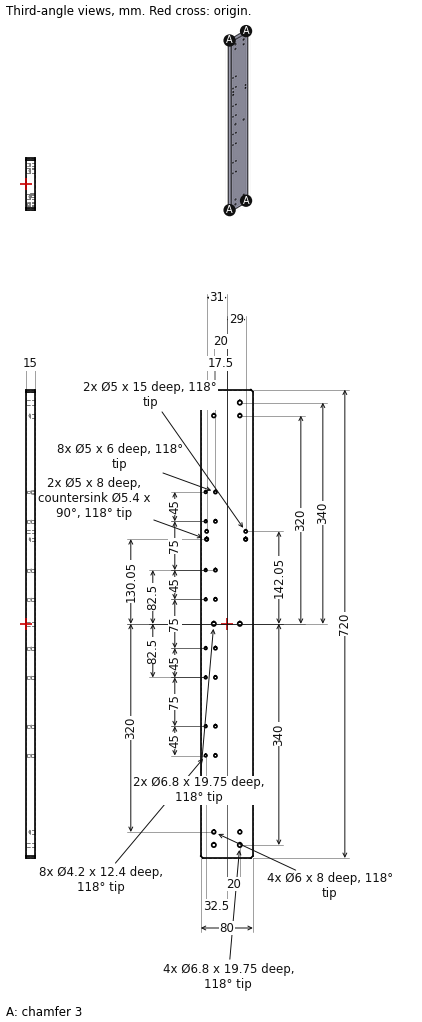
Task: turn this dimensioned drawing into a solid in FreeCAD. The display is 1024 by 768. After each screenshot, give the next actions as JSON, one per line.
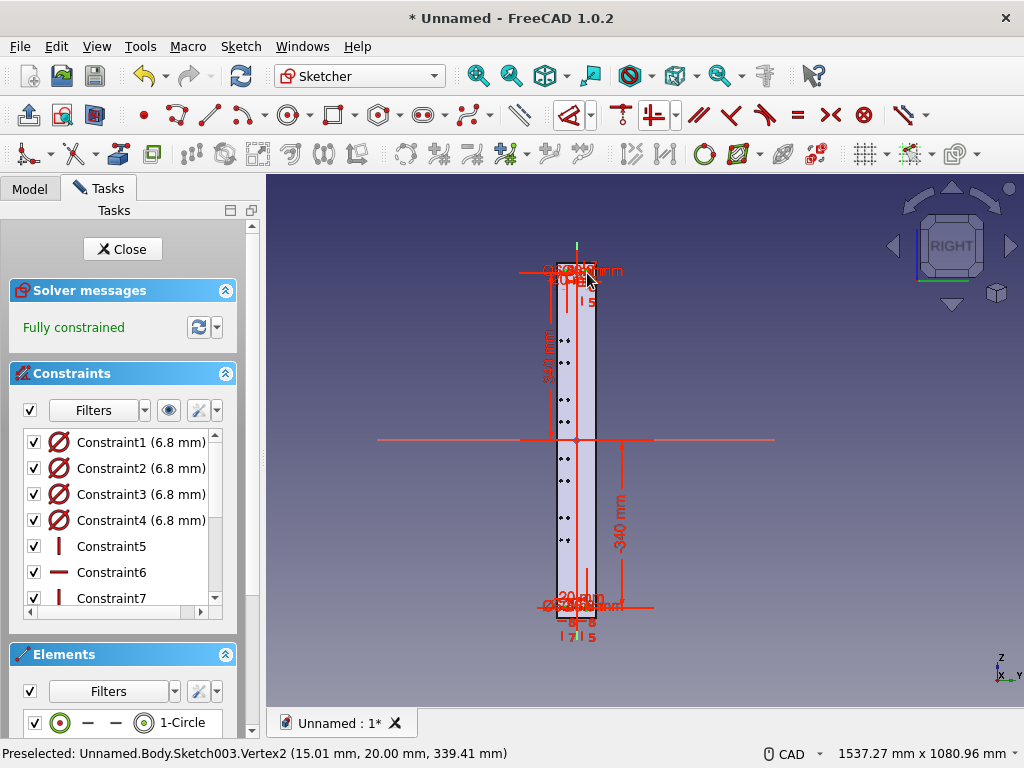
{"action": "left_click", "coordinate": [123, 249]}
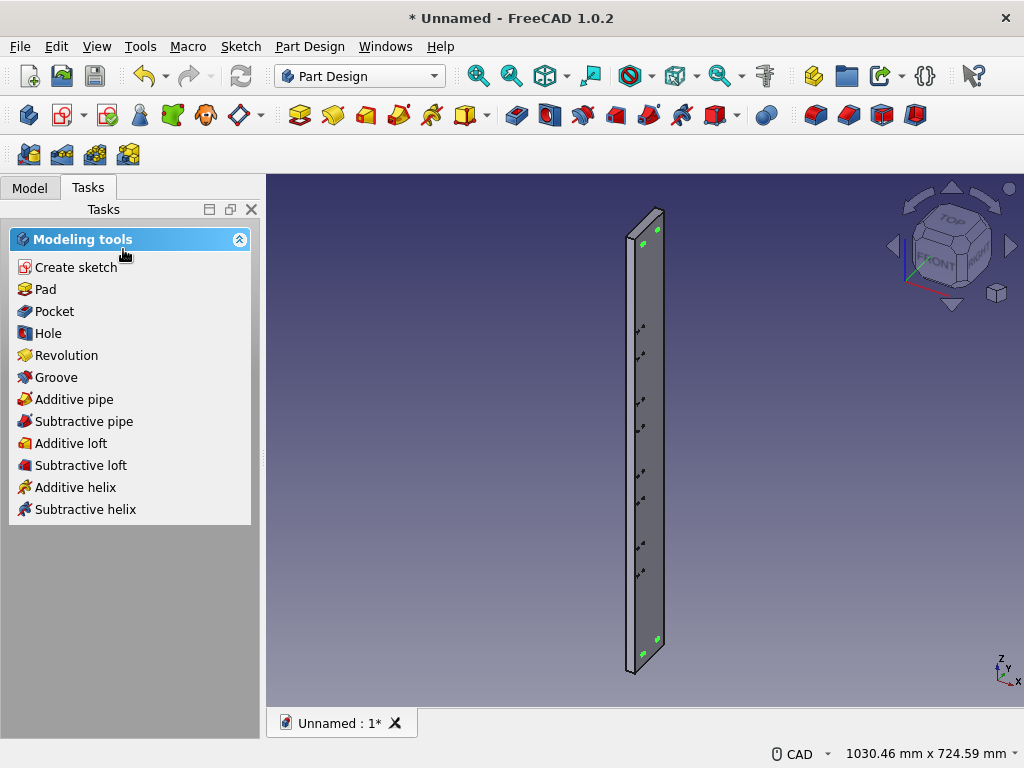
{"action": "left_click", "coordinate": [550, 116]}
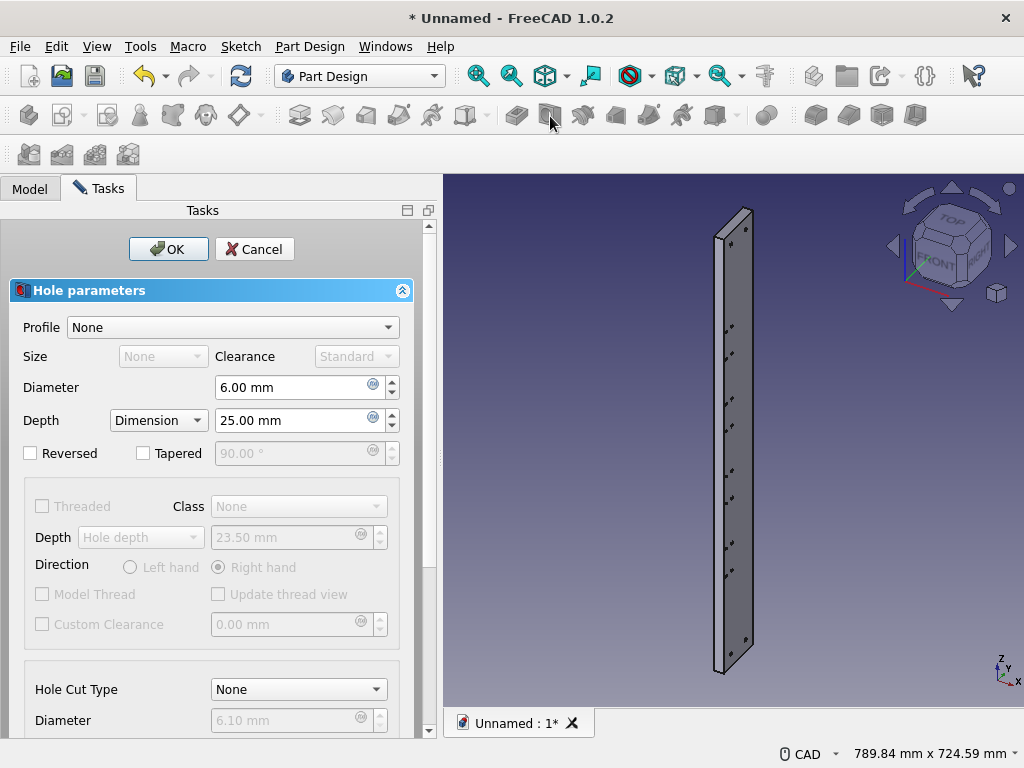
{"action": "triple_click", "coordinate": [300, 388]}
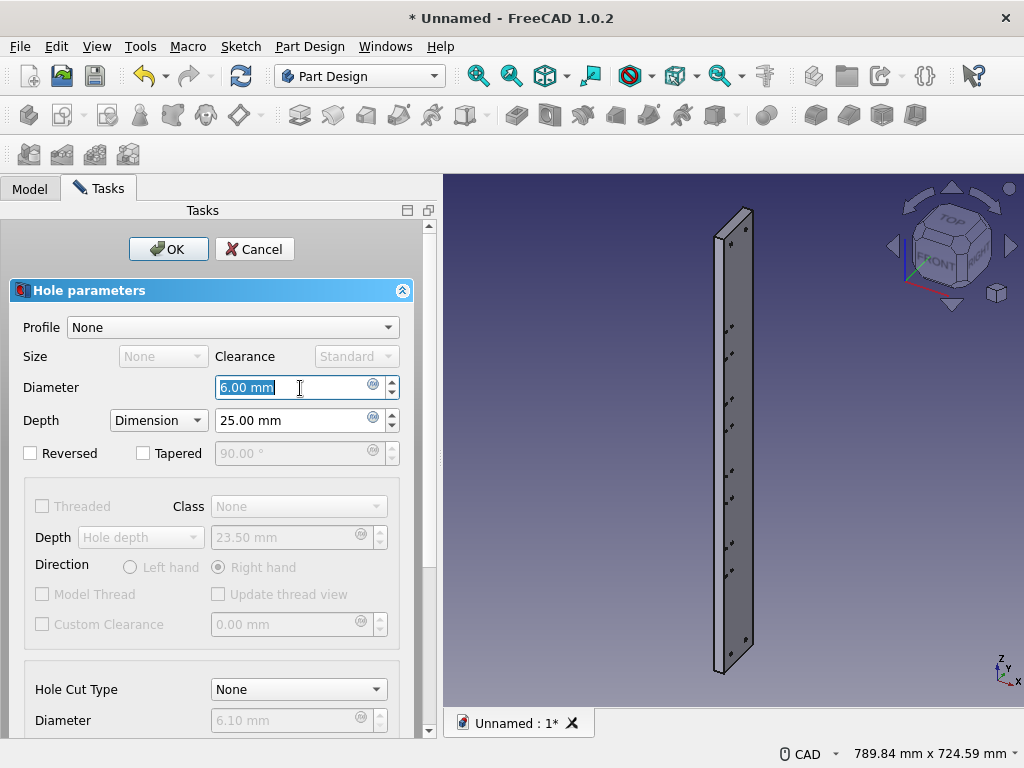
{"action": "type", "text": "6.8"}
{"action": "key", "text": "Tab"}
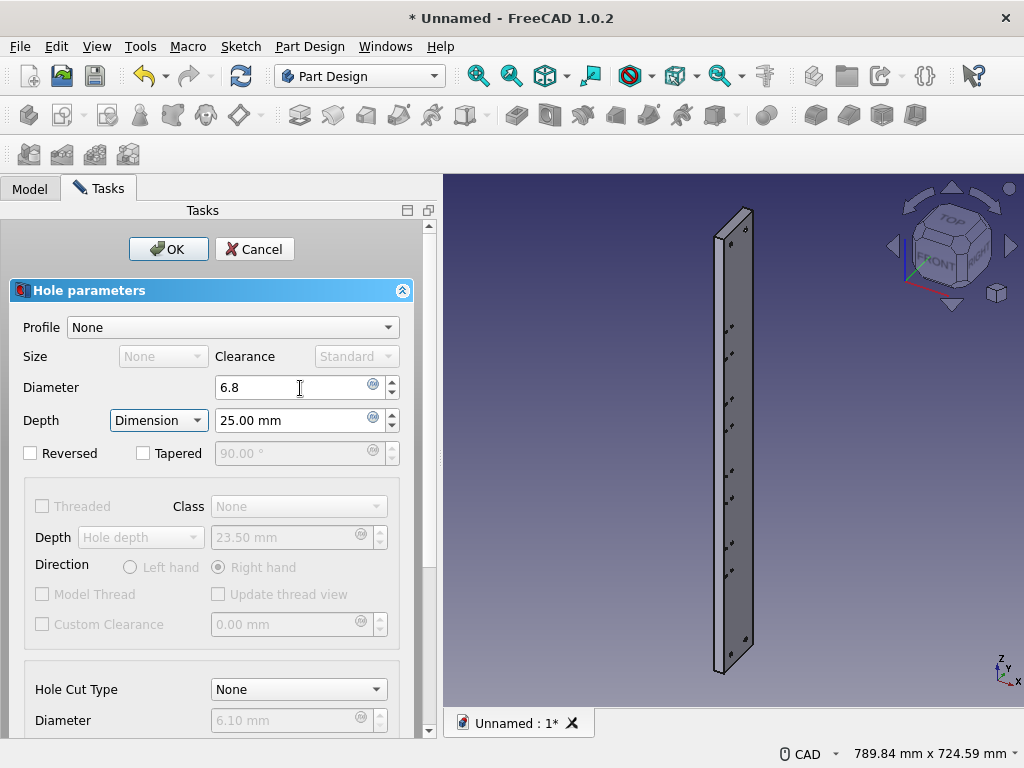
{"action": "triple_click", "coordinate": [300, 420]}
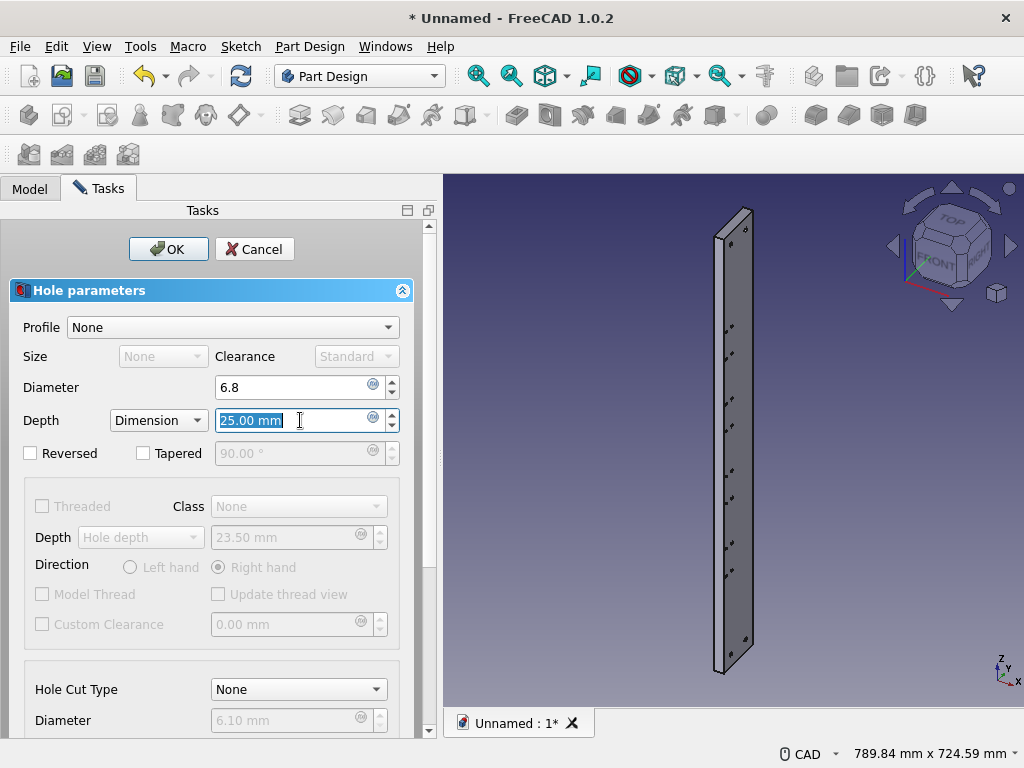
{"action": "type", "text": "19.75"}
{"action": "key", "text": "Tab"}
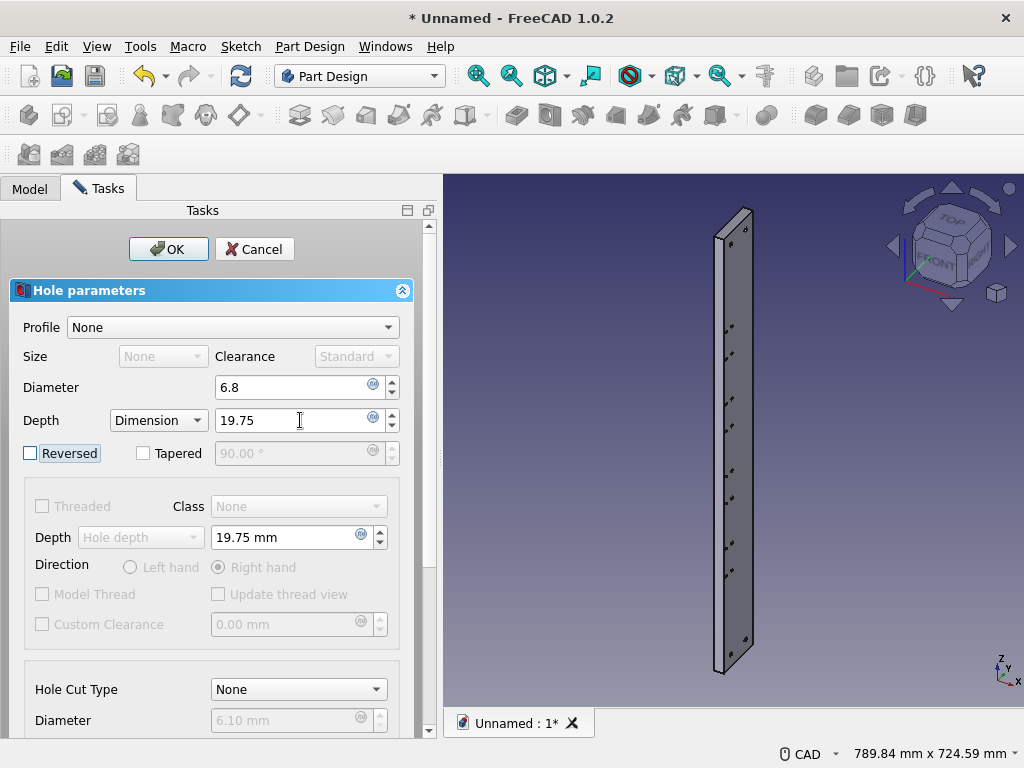
{"action": "left_click", "coordinate": [169, 249]}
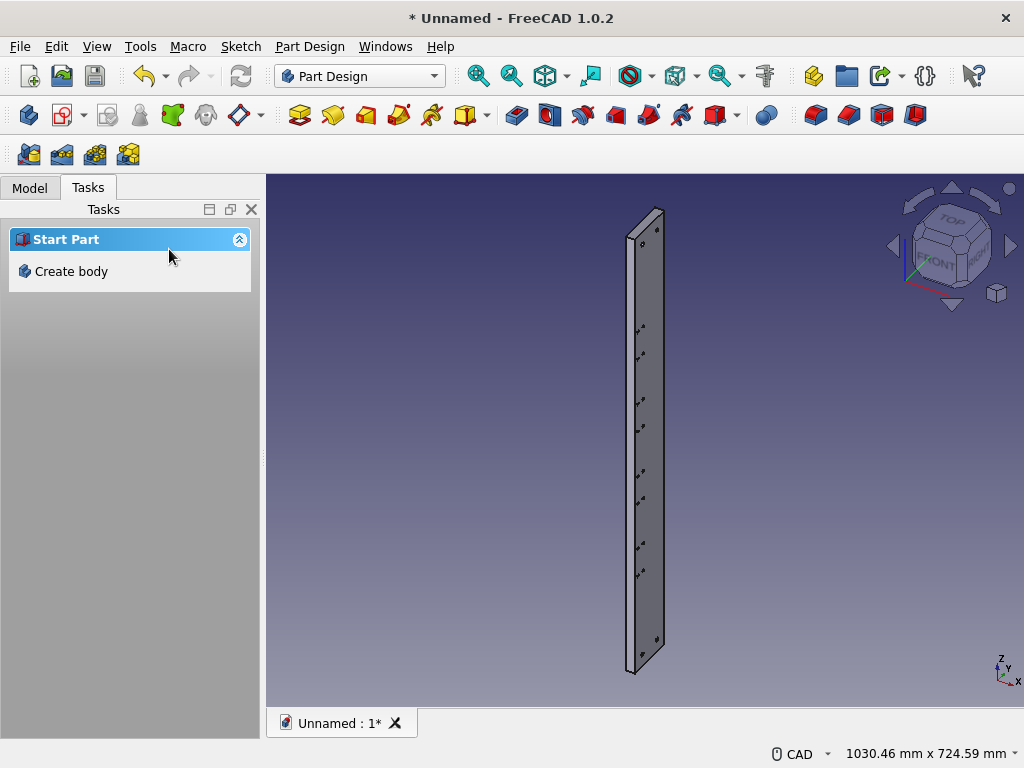
{"action": "left_click", "coordinate": [650, 441]}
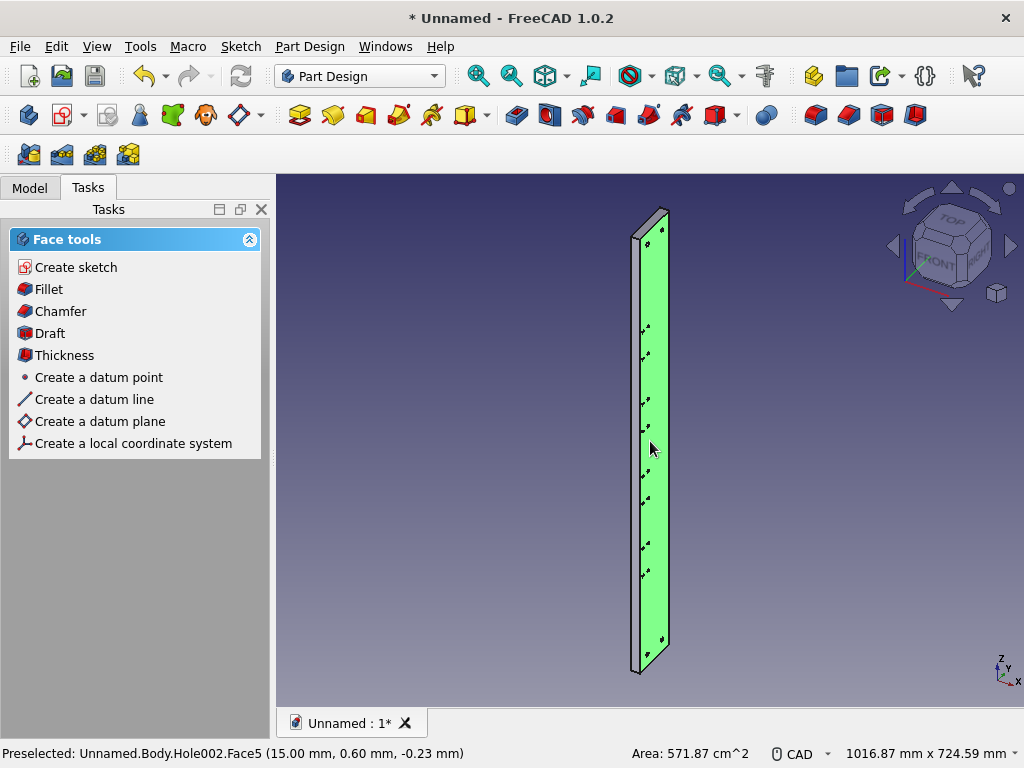
{"action": "left_click", "coordinate": [62, 116]}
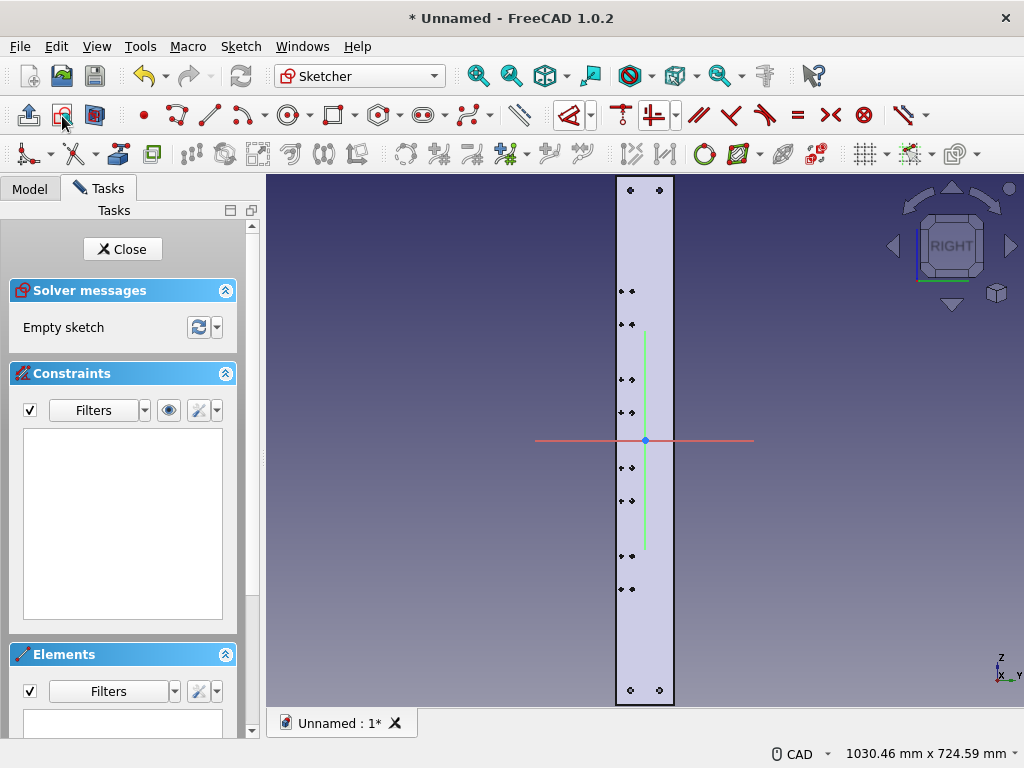
{"action": "scroll", "coordinate": [437, 440], "scroll_direction": "down", "scroll_amount": 2}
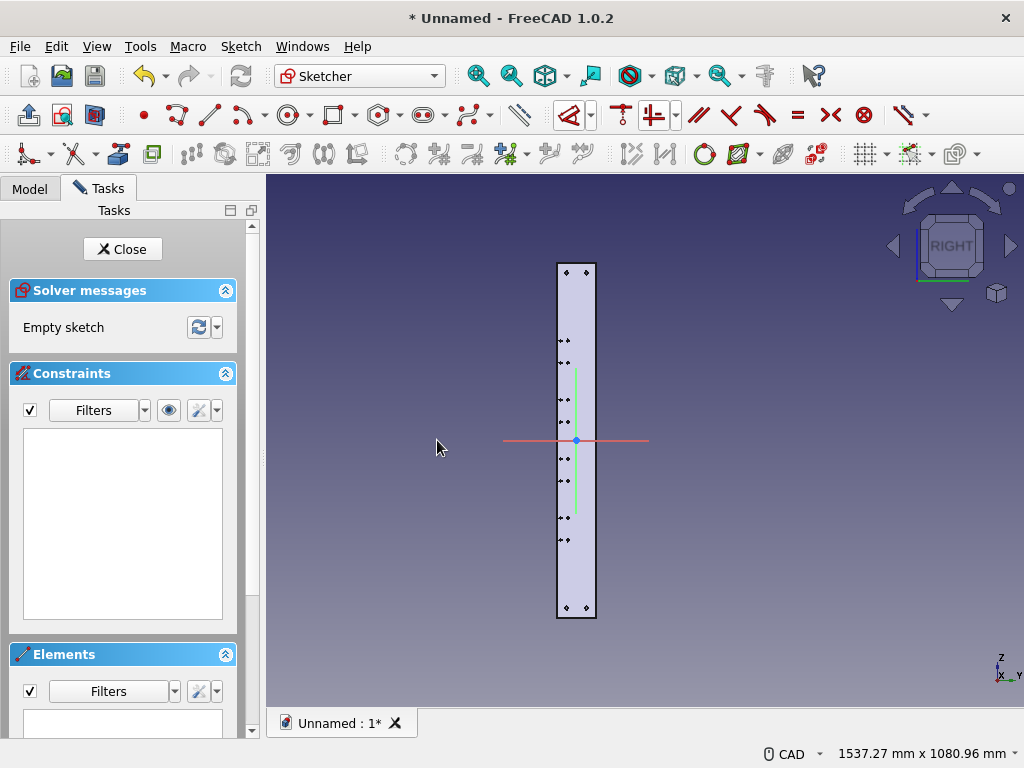
{"action": "left_click", "coordinate": [288, 116]}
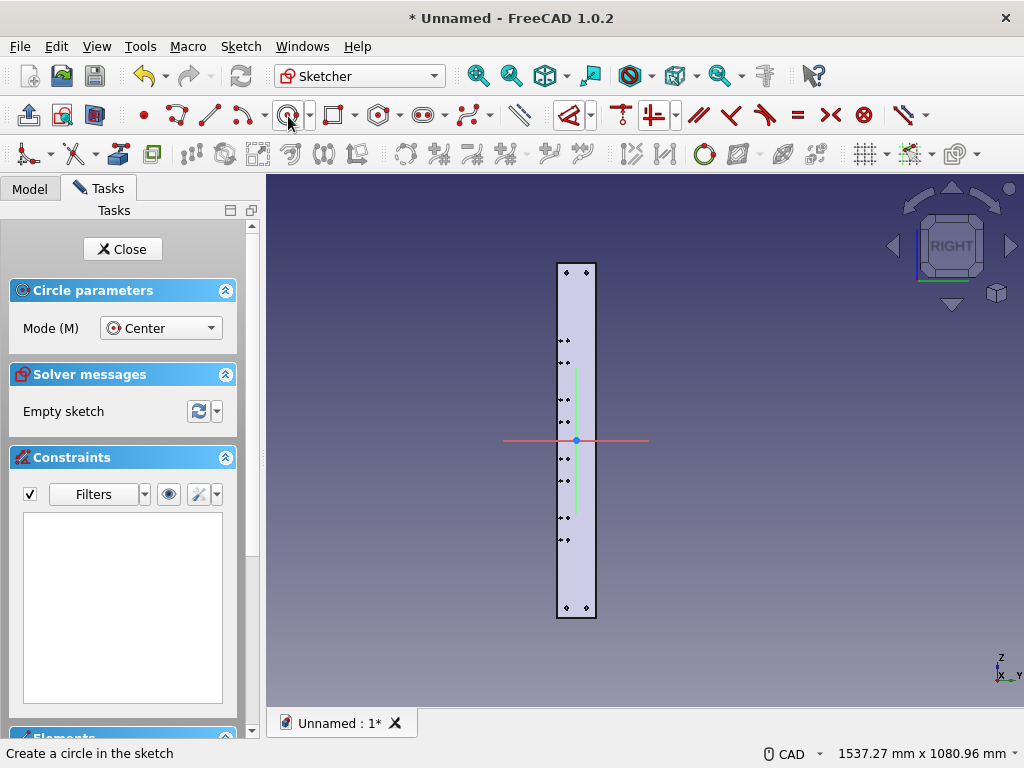
{"action": "scroll", "coordinate": [567, 598], "scroll_direction": "up", "scroll_amount": 14}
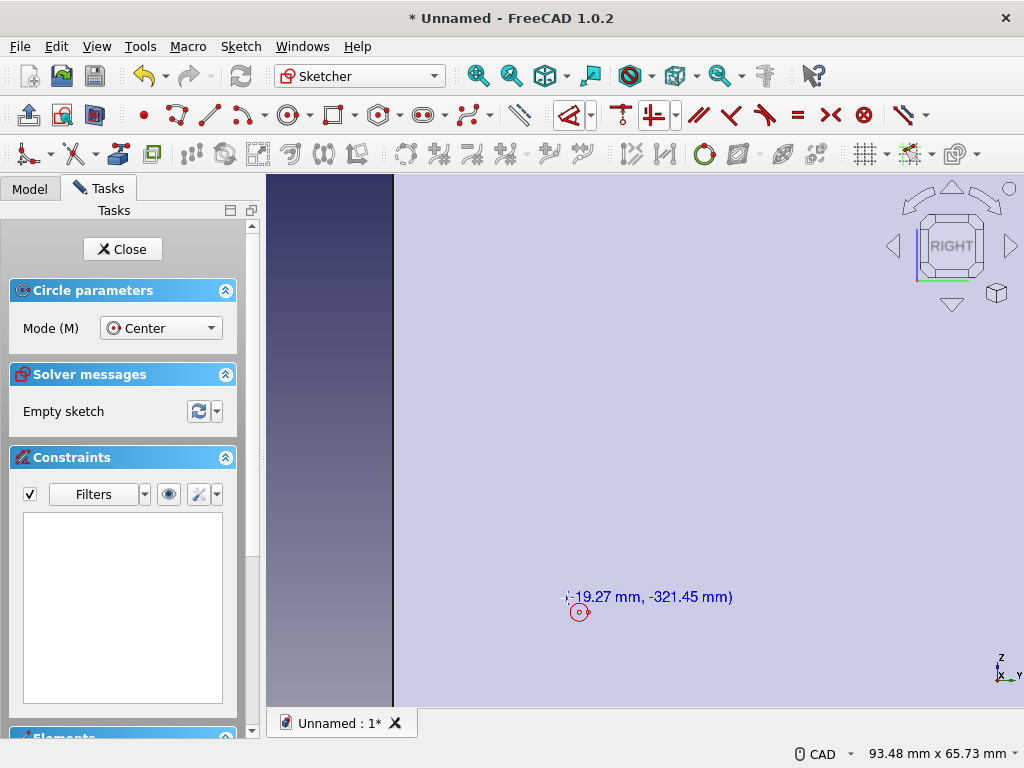
{"action": "scroll", "coordinate": [567, 599], "scroll_direction": "down", "scroll_amount": 14}